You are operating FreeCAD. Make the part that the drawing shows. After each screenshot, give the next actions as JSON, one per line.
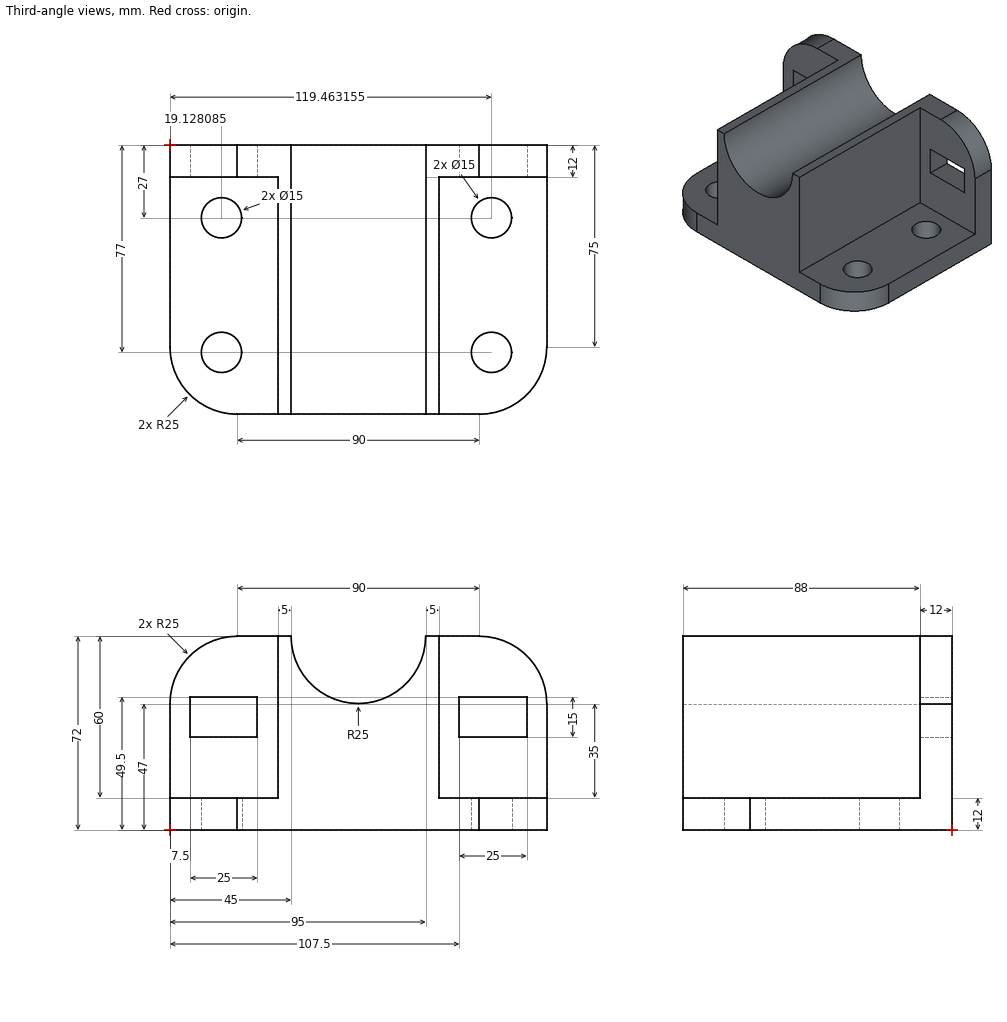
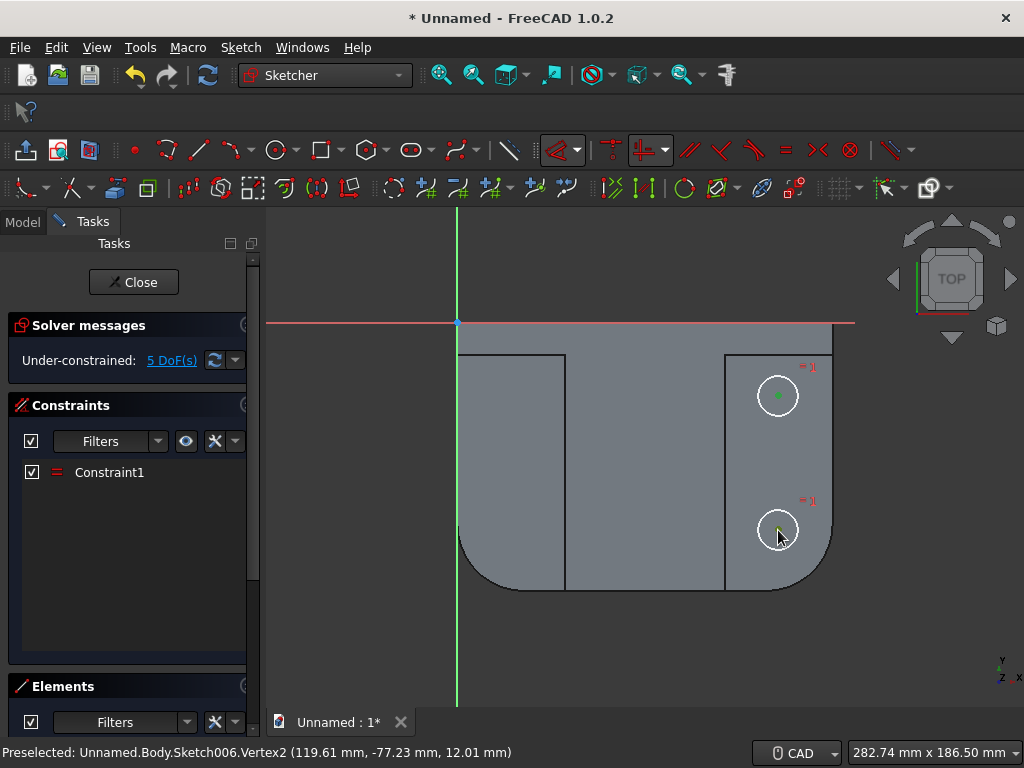
{"action": "key", "text": "v"}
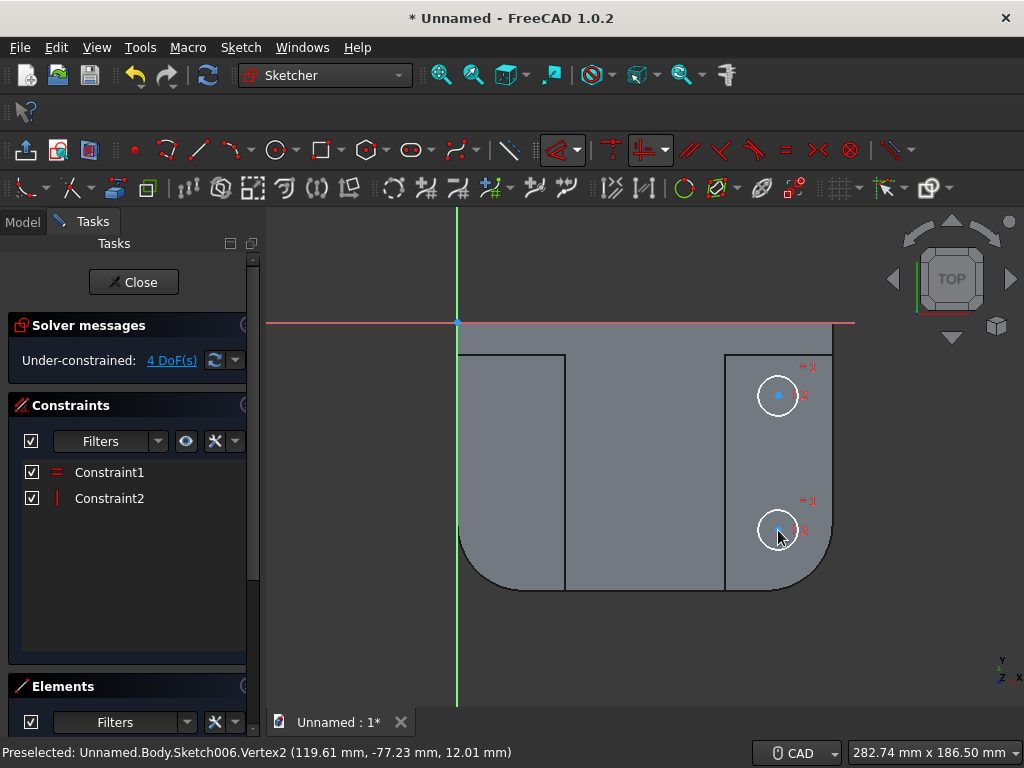
{"action": "left_click", "coordinate": [792, 382]}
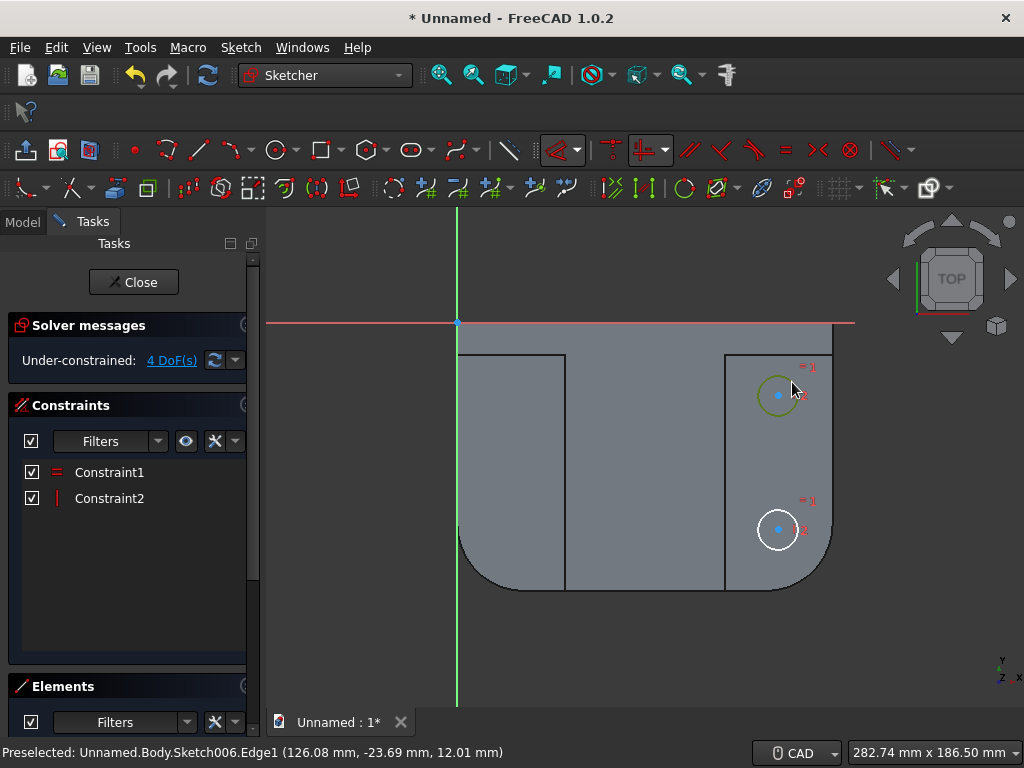
{"action": "key", "text": "k o"}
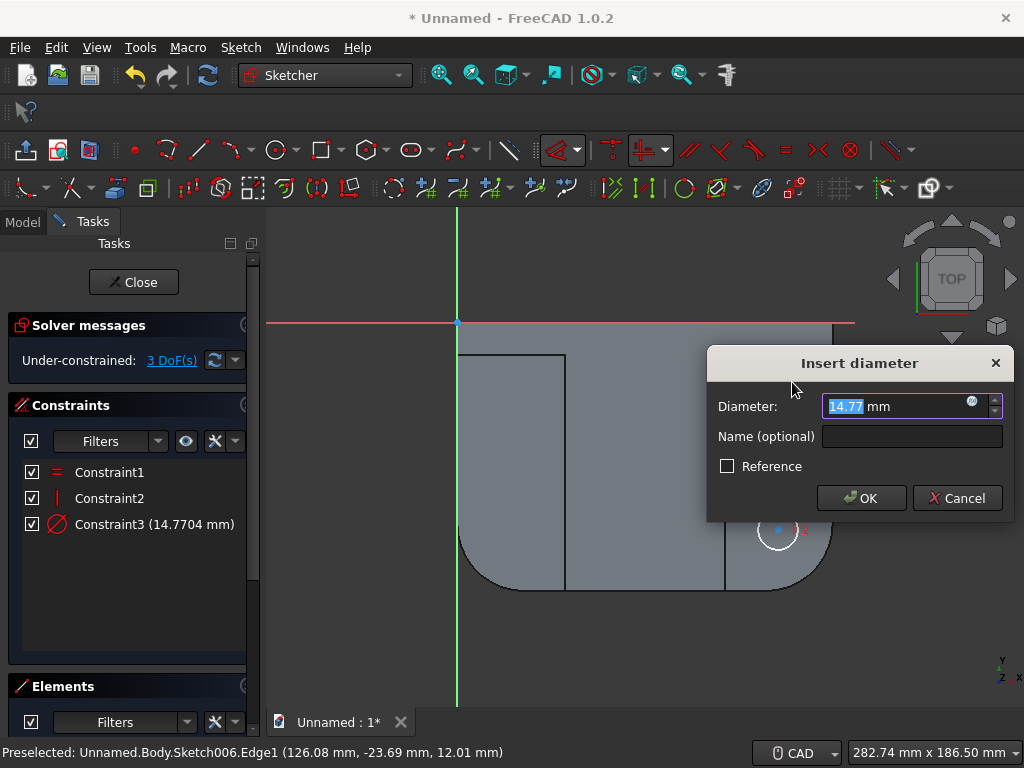
{"action": "type", "text": "15"}
{"action": "key", "text": "Return"}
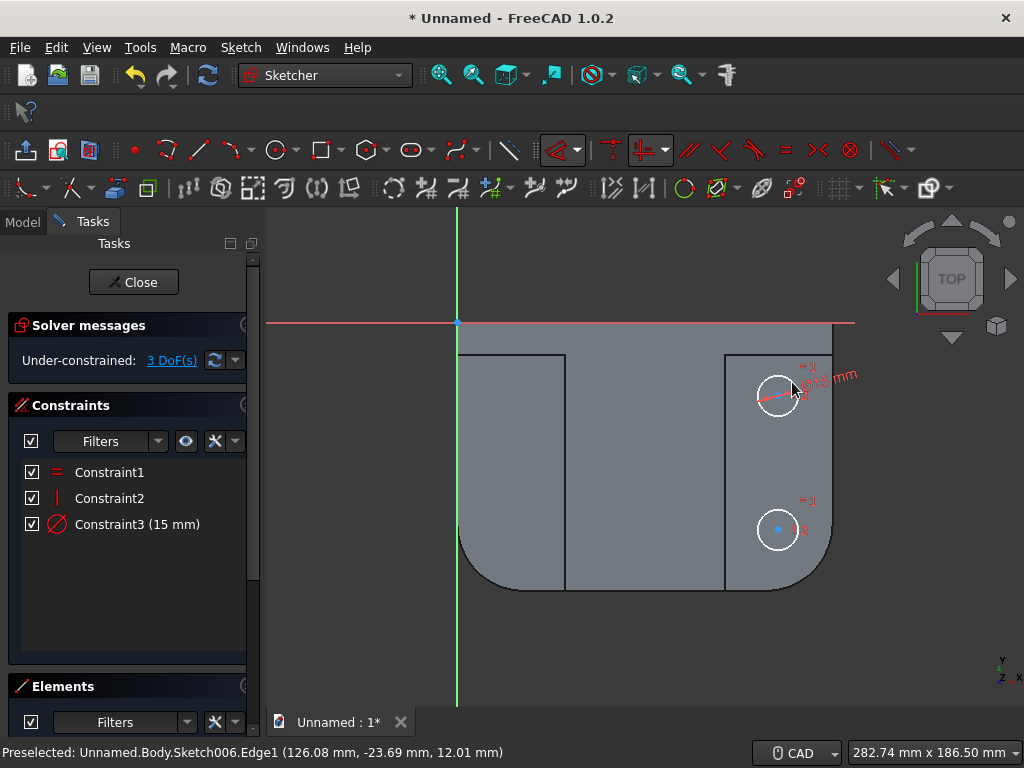
{"action": "left_click", "coordinate": [778, 396]}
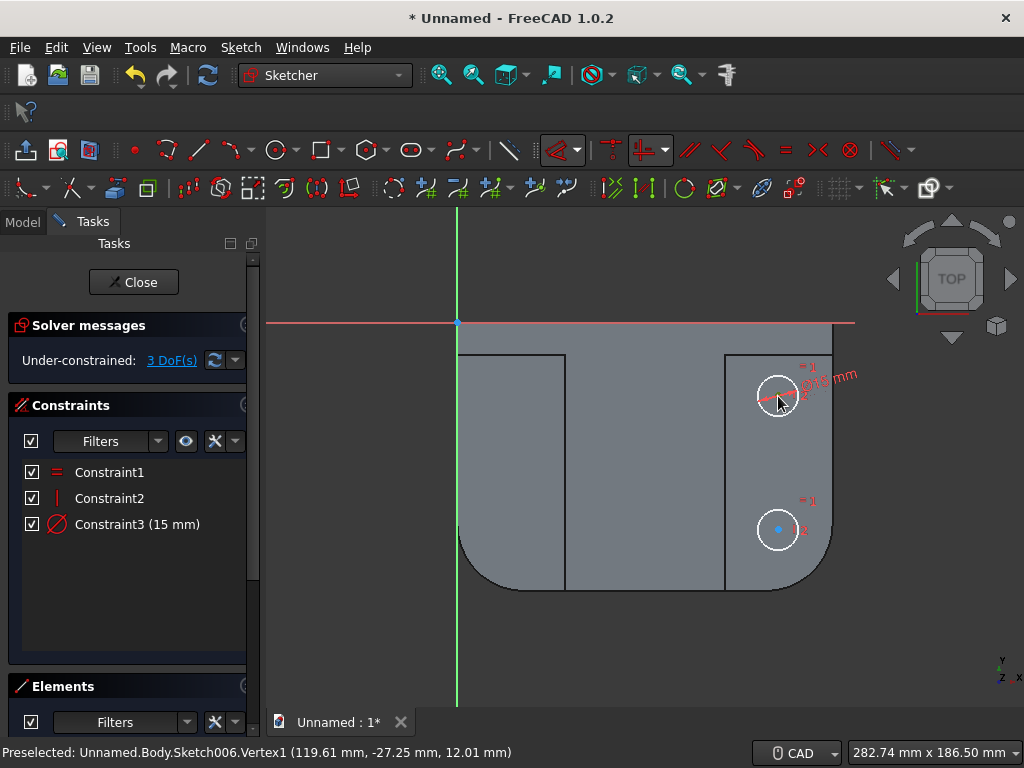
{"action": "key", "text": "i"}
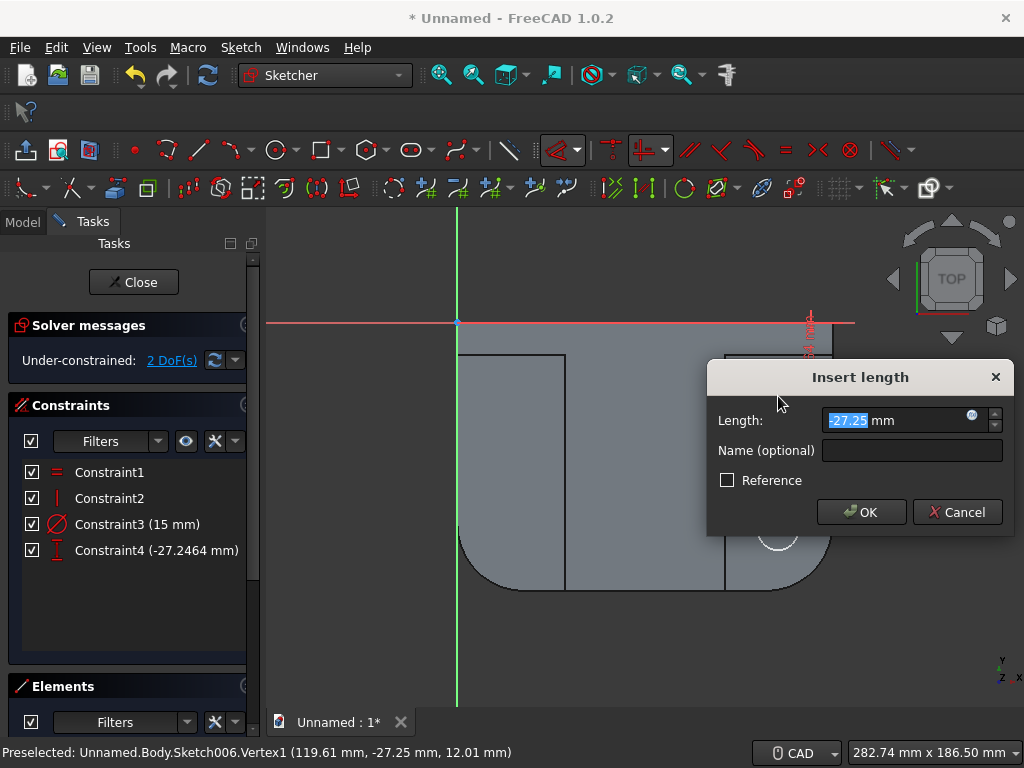
{"action": "type", "text": "-27"}
{"action": "key", "text": "Return"}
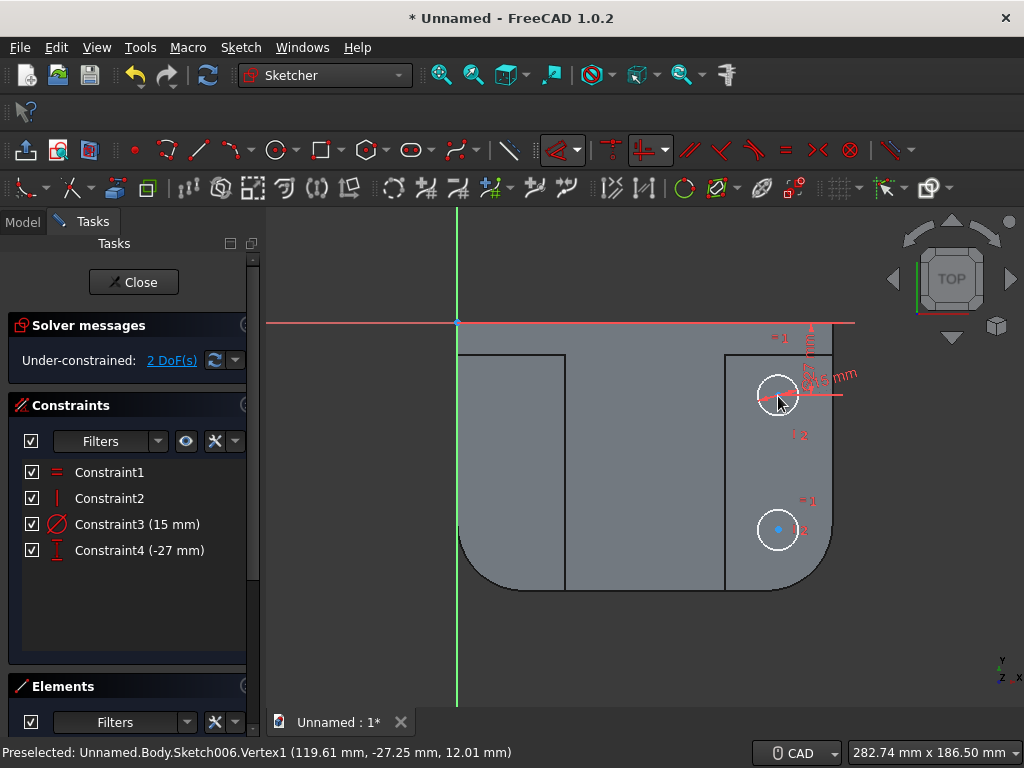
{"action": "left_click", "coordinate": [778, 530]}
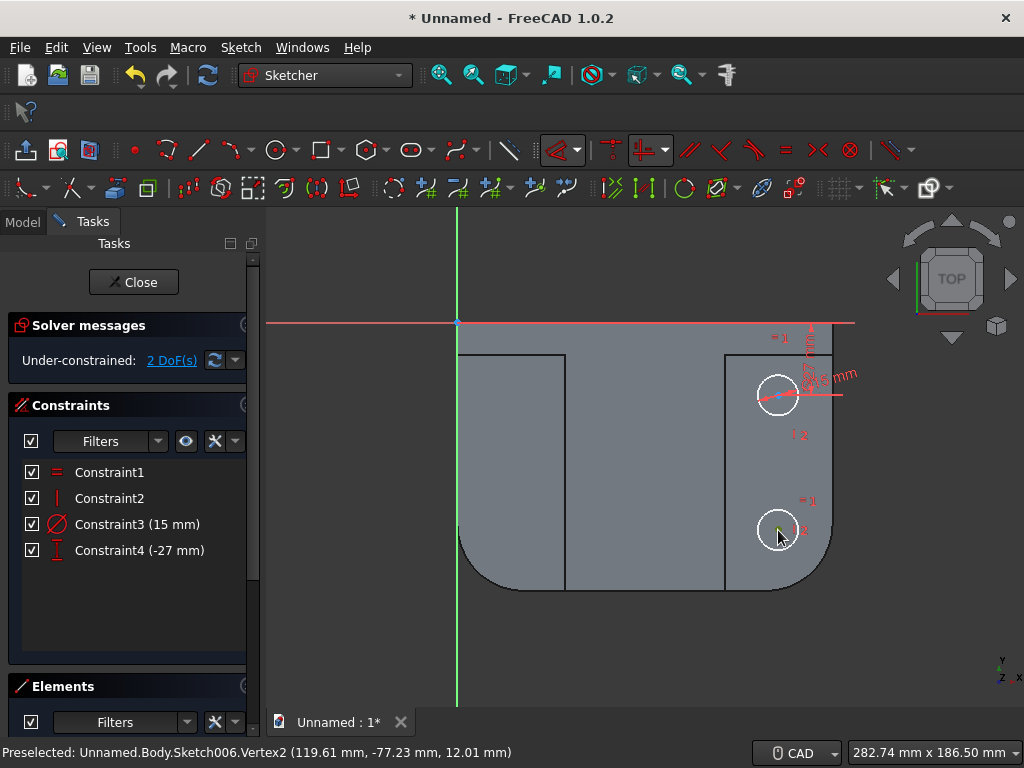
{"action": "key", "text": "i"}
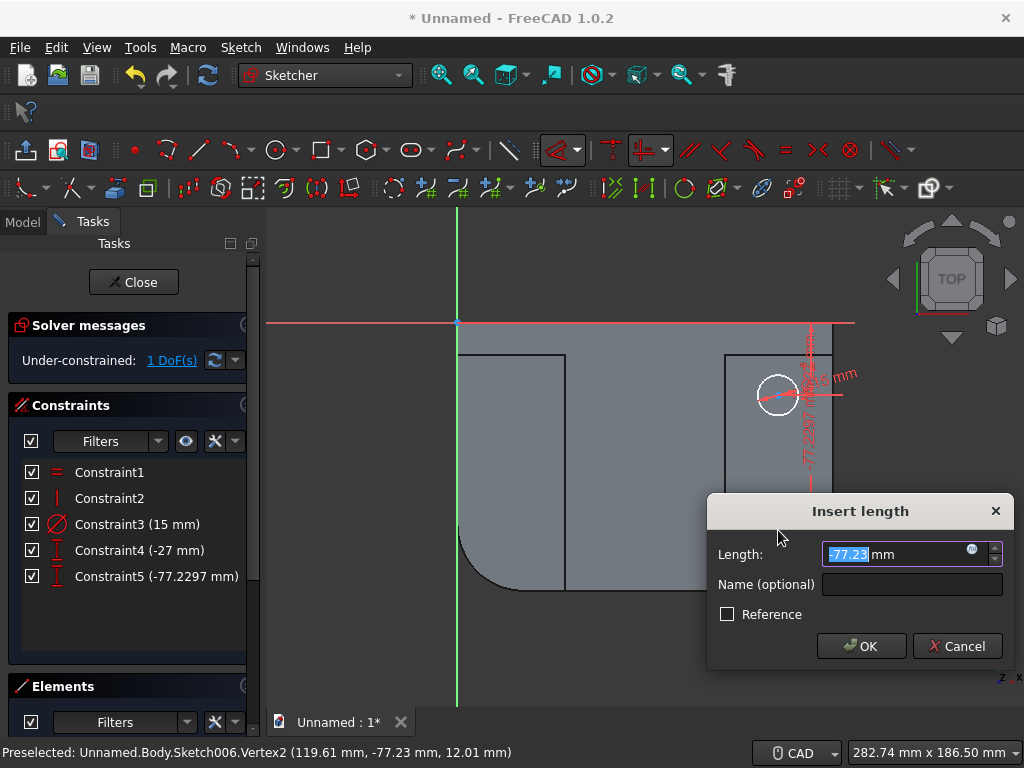
{"action": "type", "text": "-77"}
{"action": "key", "text": "Return"}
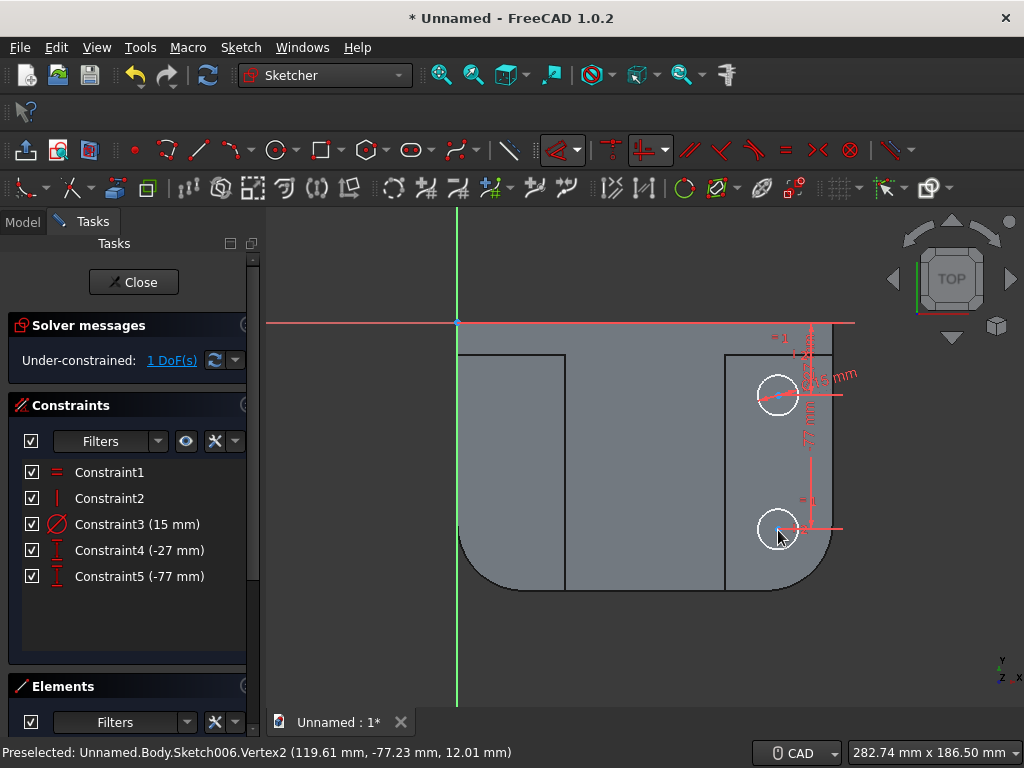
{"action": "left_click", "coordinate": [778, 395]}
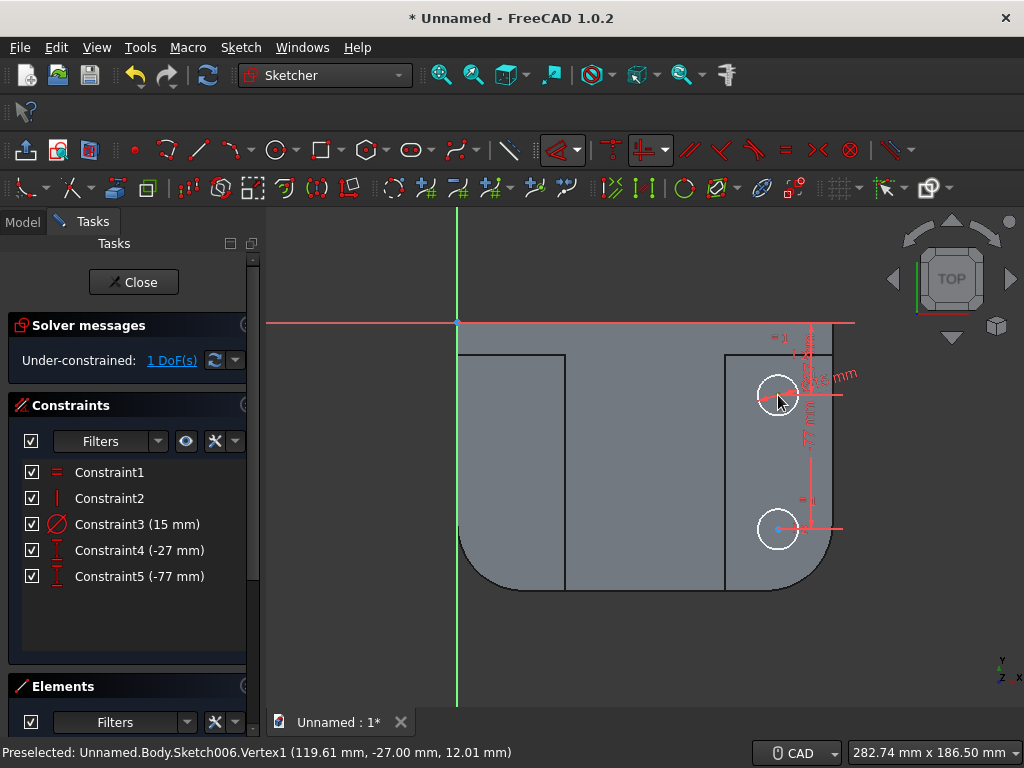
{"action": "key", "text": "l"}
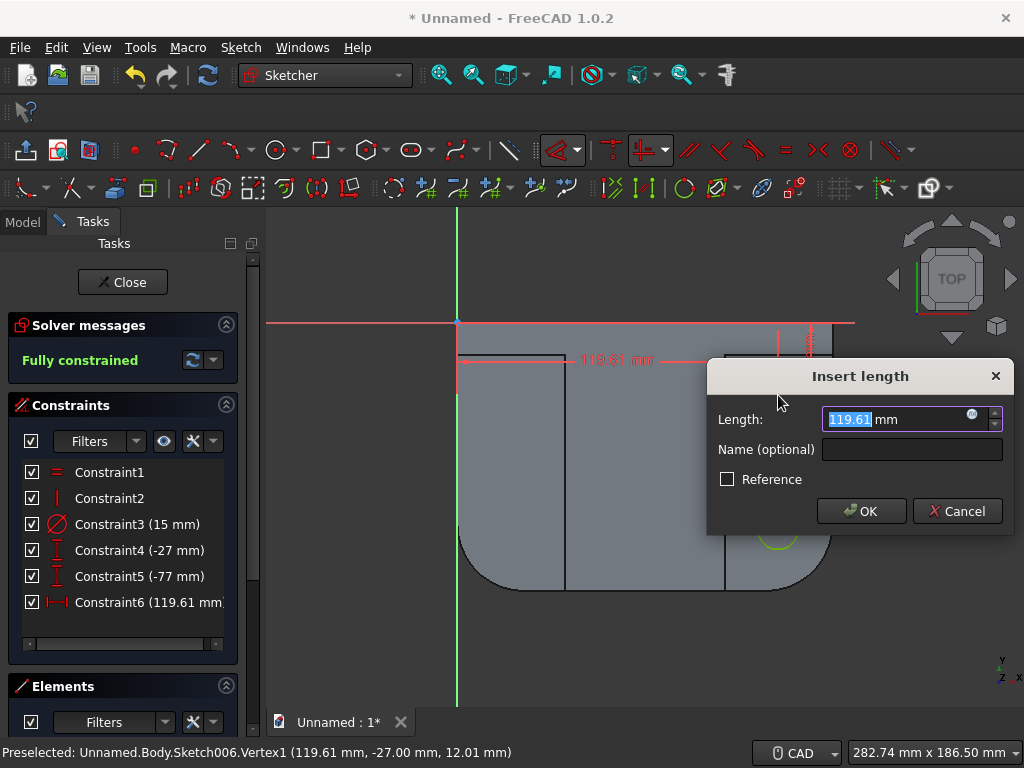
{"action": "type", "text": "119.463155"}
{"action": "key", "text": "Return"}